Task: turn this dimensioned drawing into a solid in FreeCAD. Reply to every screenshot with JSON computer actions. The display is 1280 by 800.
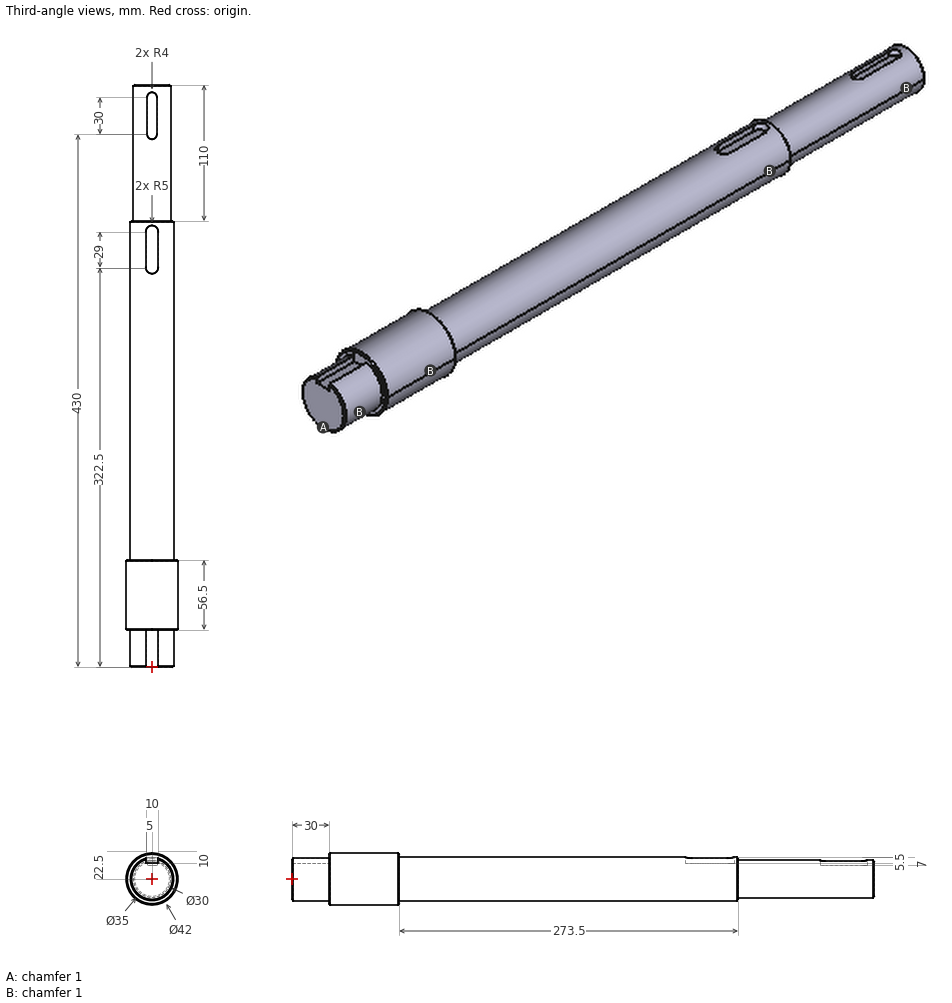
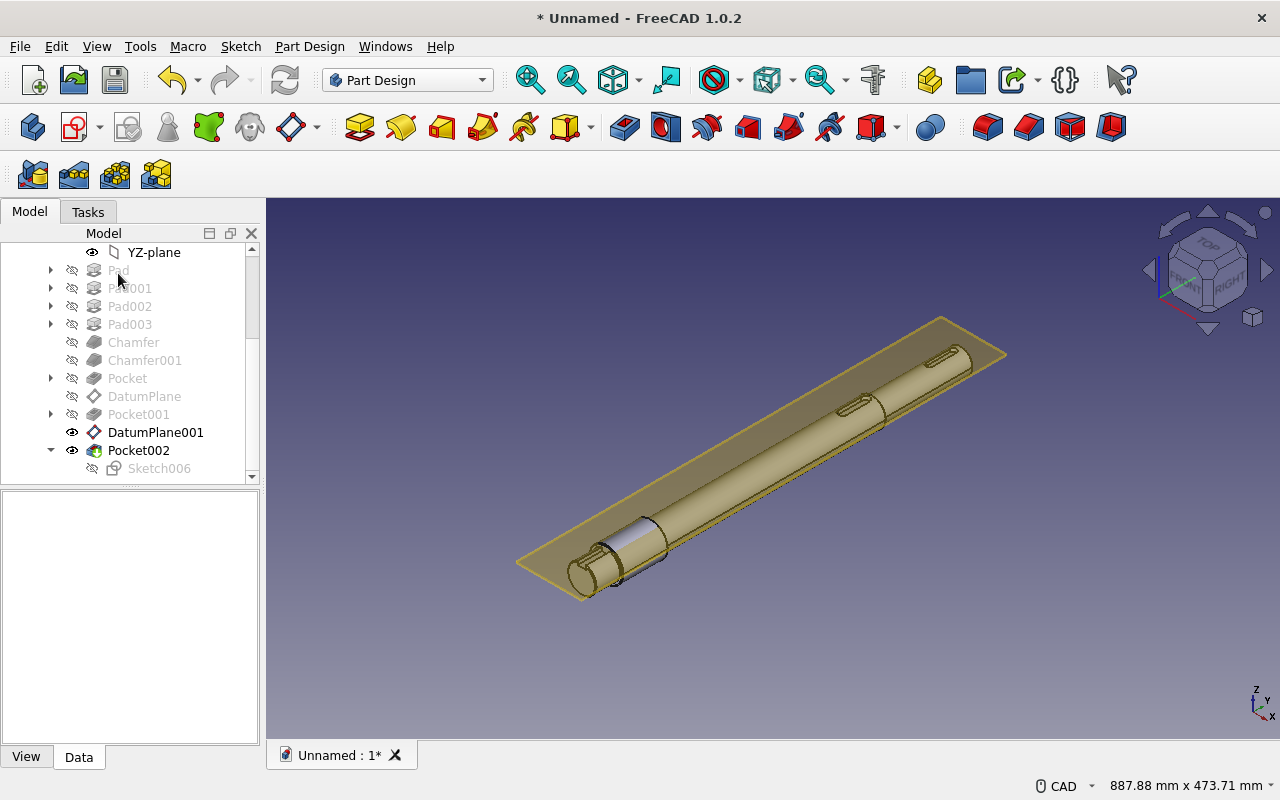
{"action": "left_click", "coordinate": [117, 432]}
{"action": "key", "text": "space"}